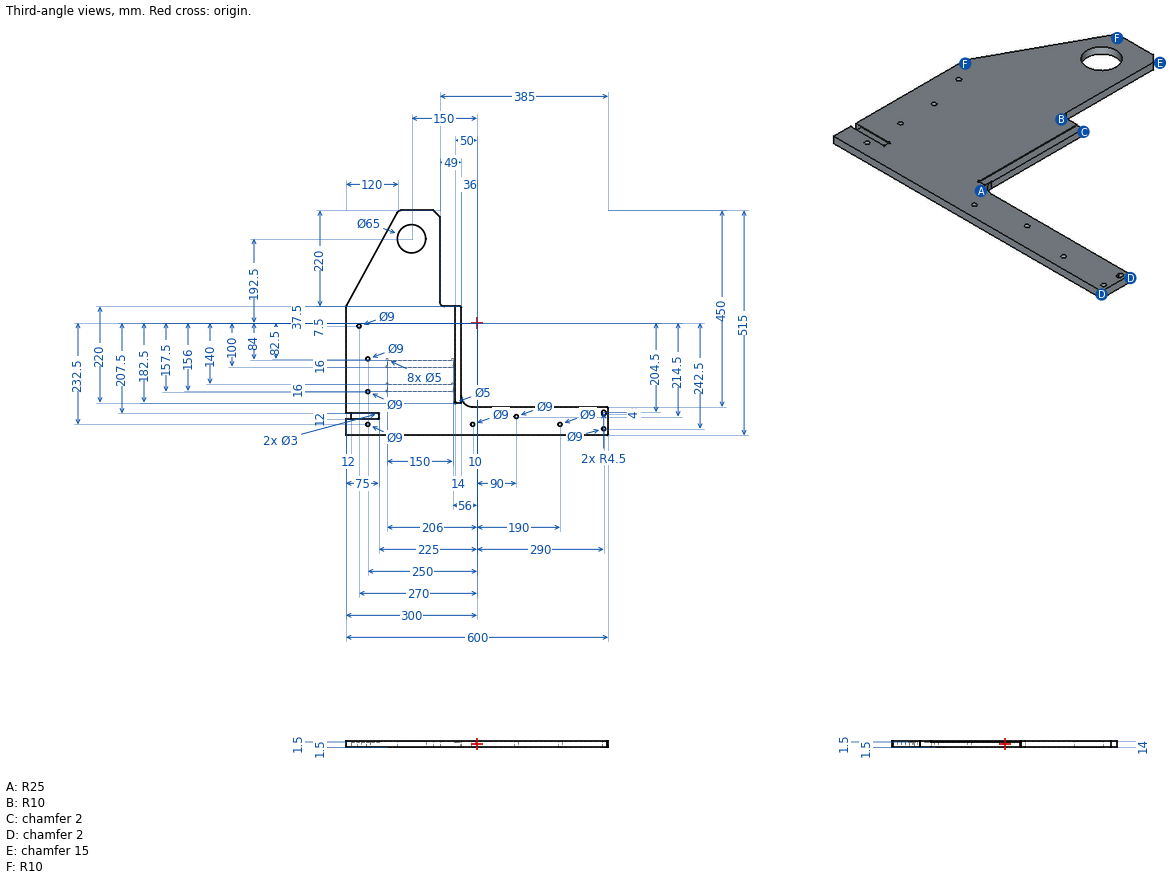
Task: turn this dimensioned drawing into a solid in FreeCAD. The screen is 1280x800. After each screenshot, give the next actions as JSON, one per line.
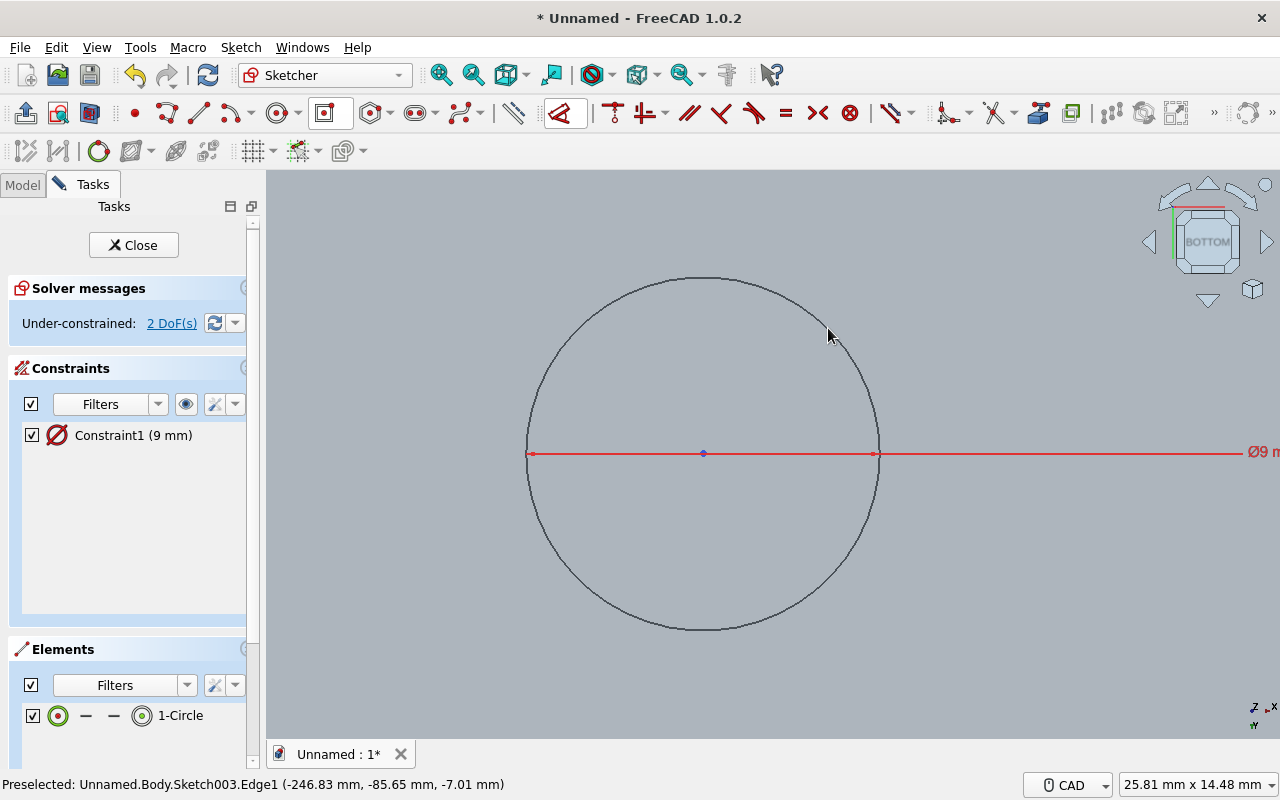
{"action": "left_click", "coordinate": [703, 454]}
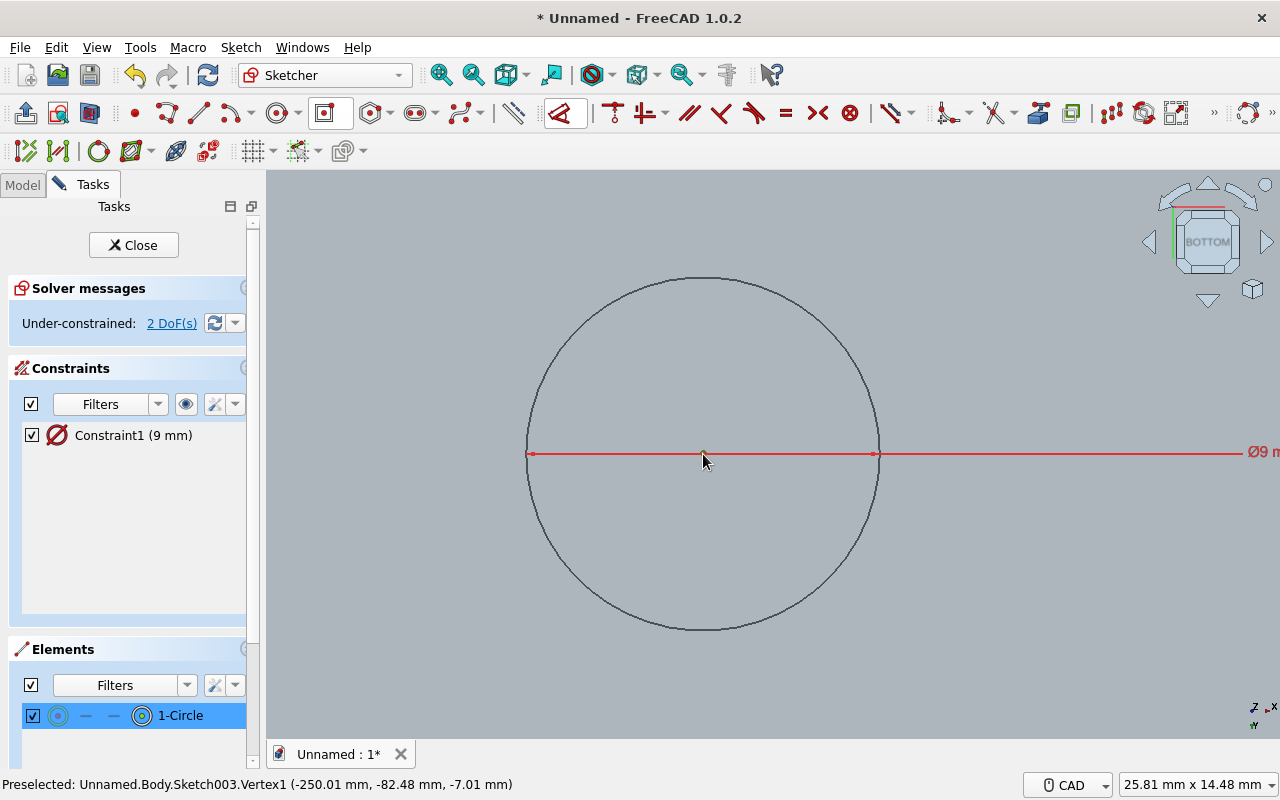
{"action": "left_click", "coordinate": [582, 114]}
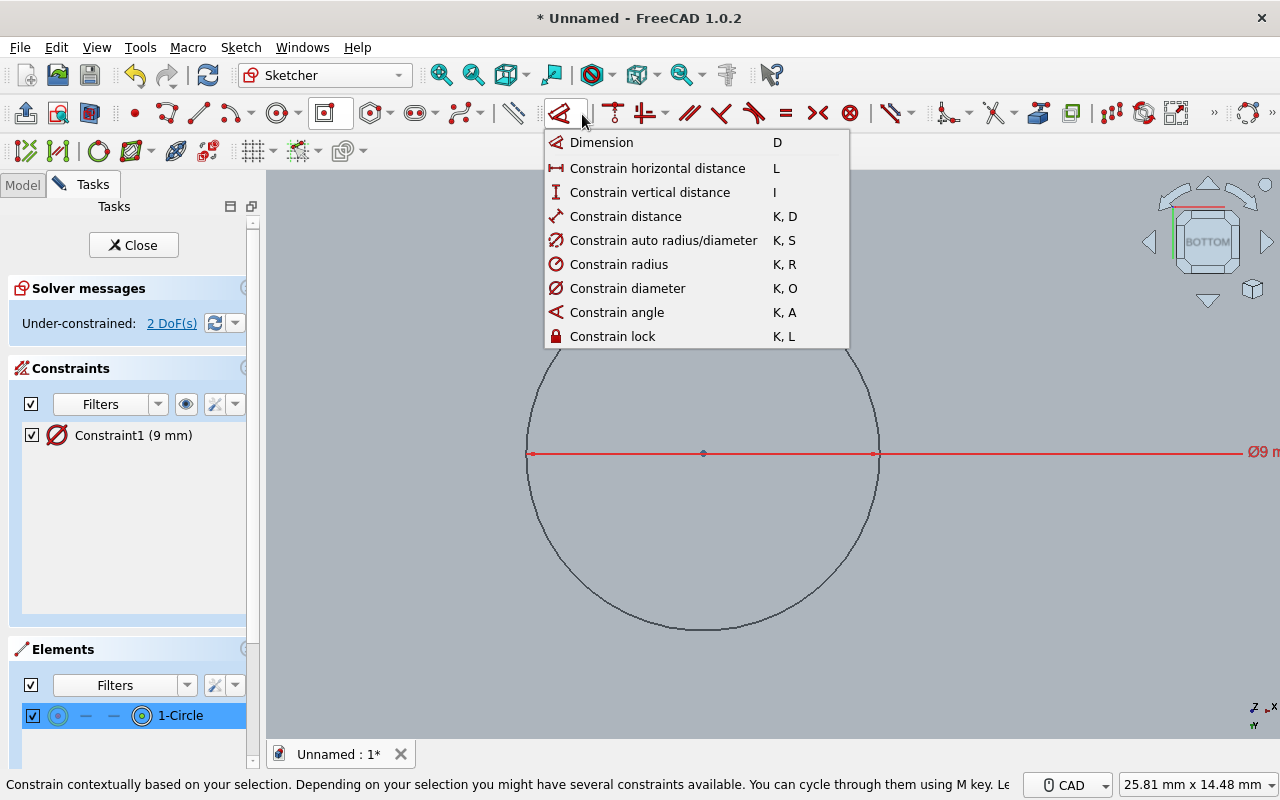
{"action": "left_click", "coordinate": [697, 168]}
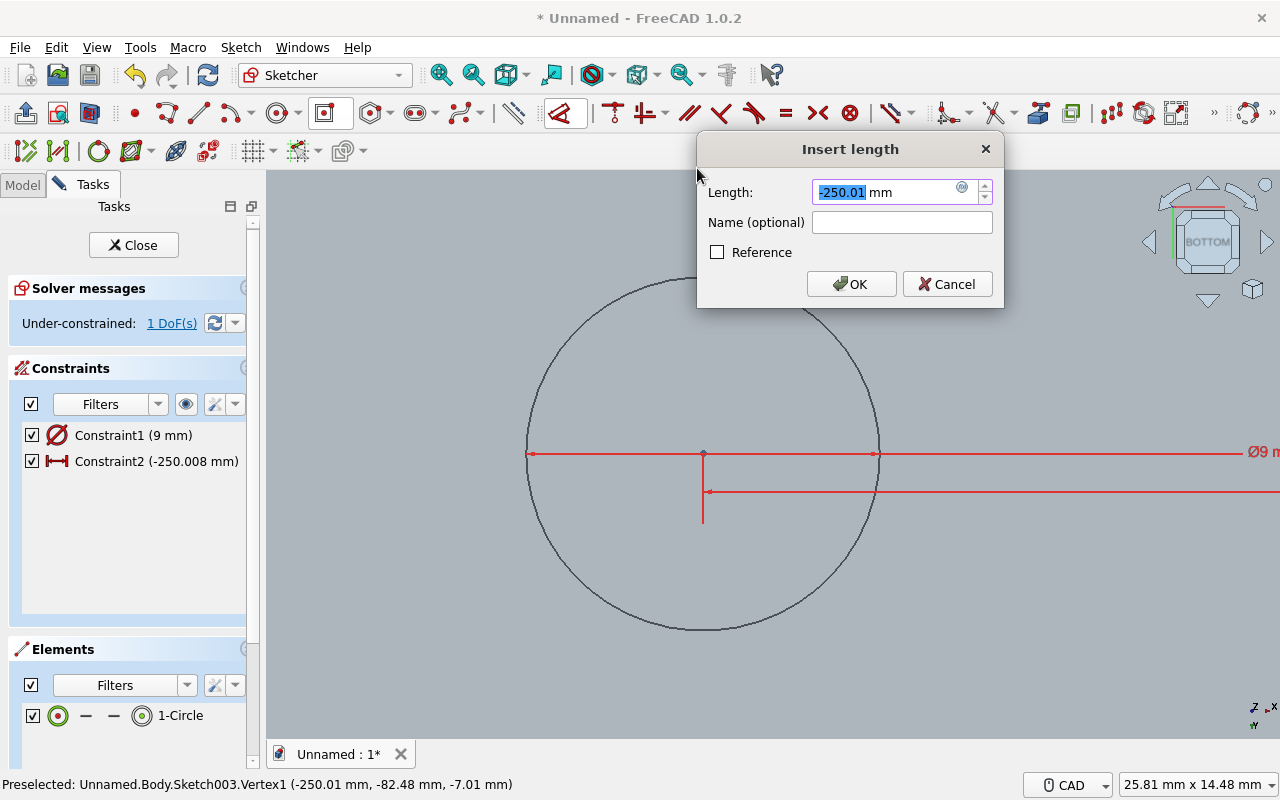
{"action": "type", "text": "-250"}
{"action": "key", "text": "Return"}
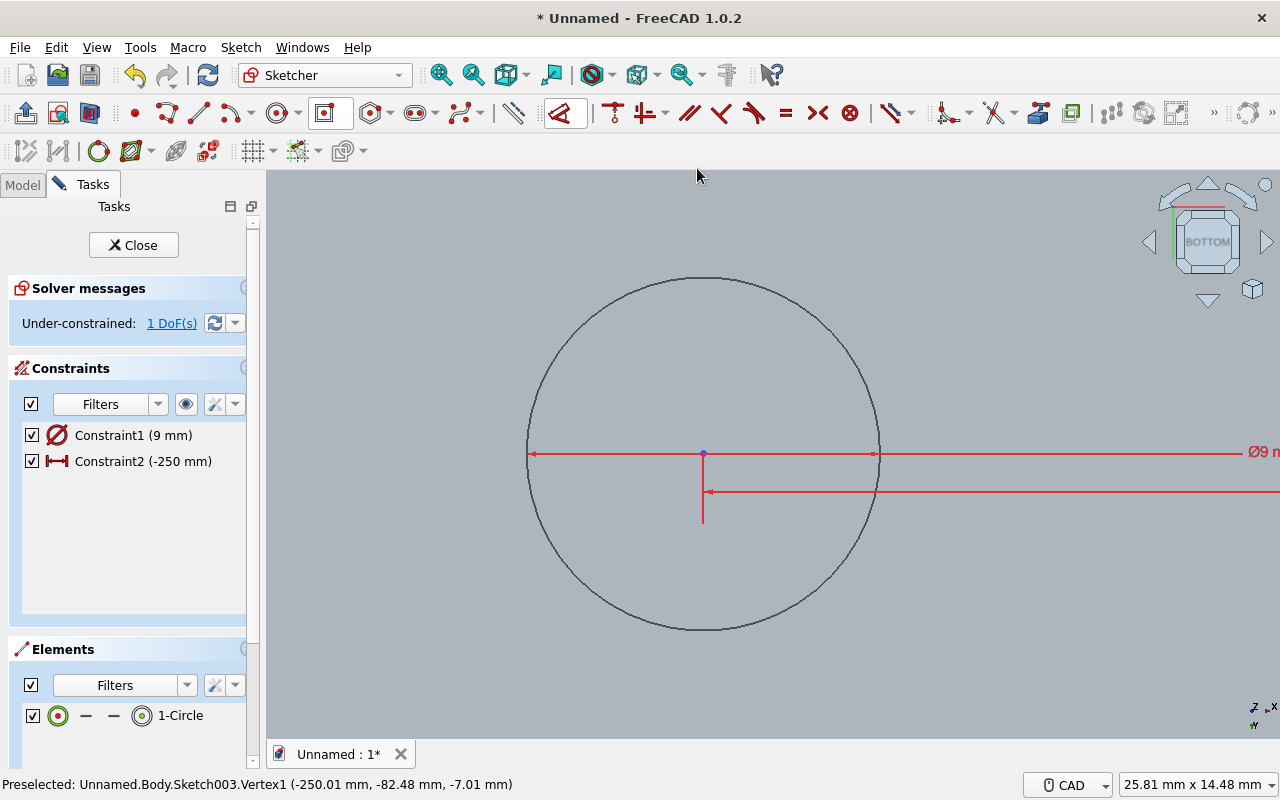
{"action": "left_click", "coordinate": [703, 454]}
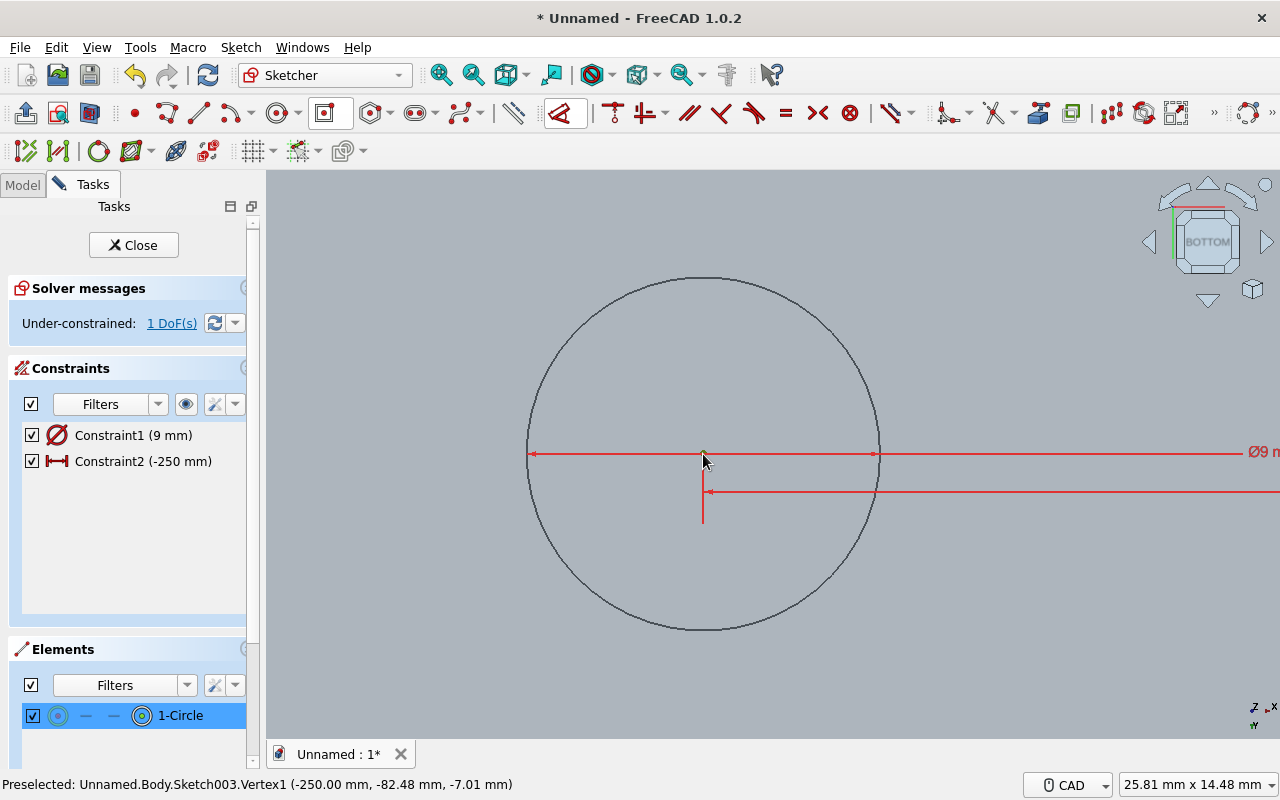
{"action": "key", "text": "i"}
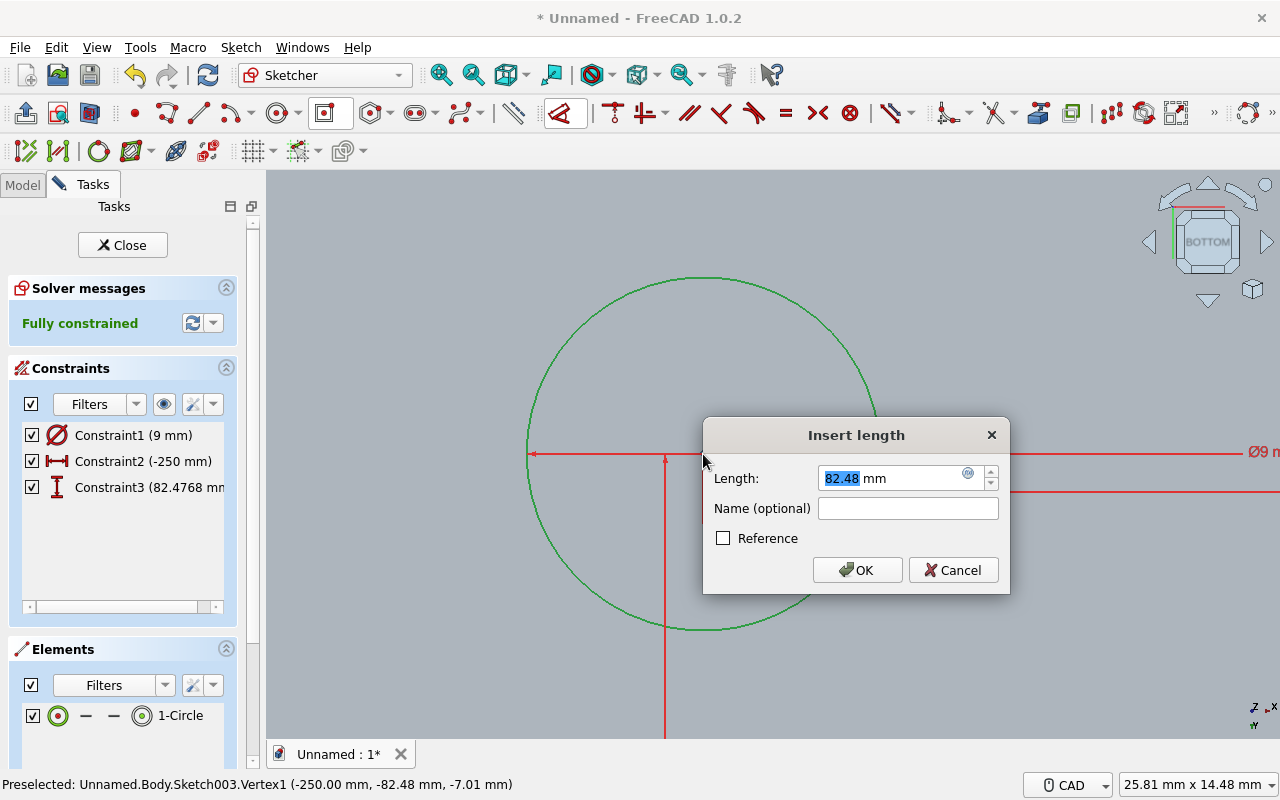
{"action": "type", "text": "82.5"}
{"action": "key", "text": "Return"}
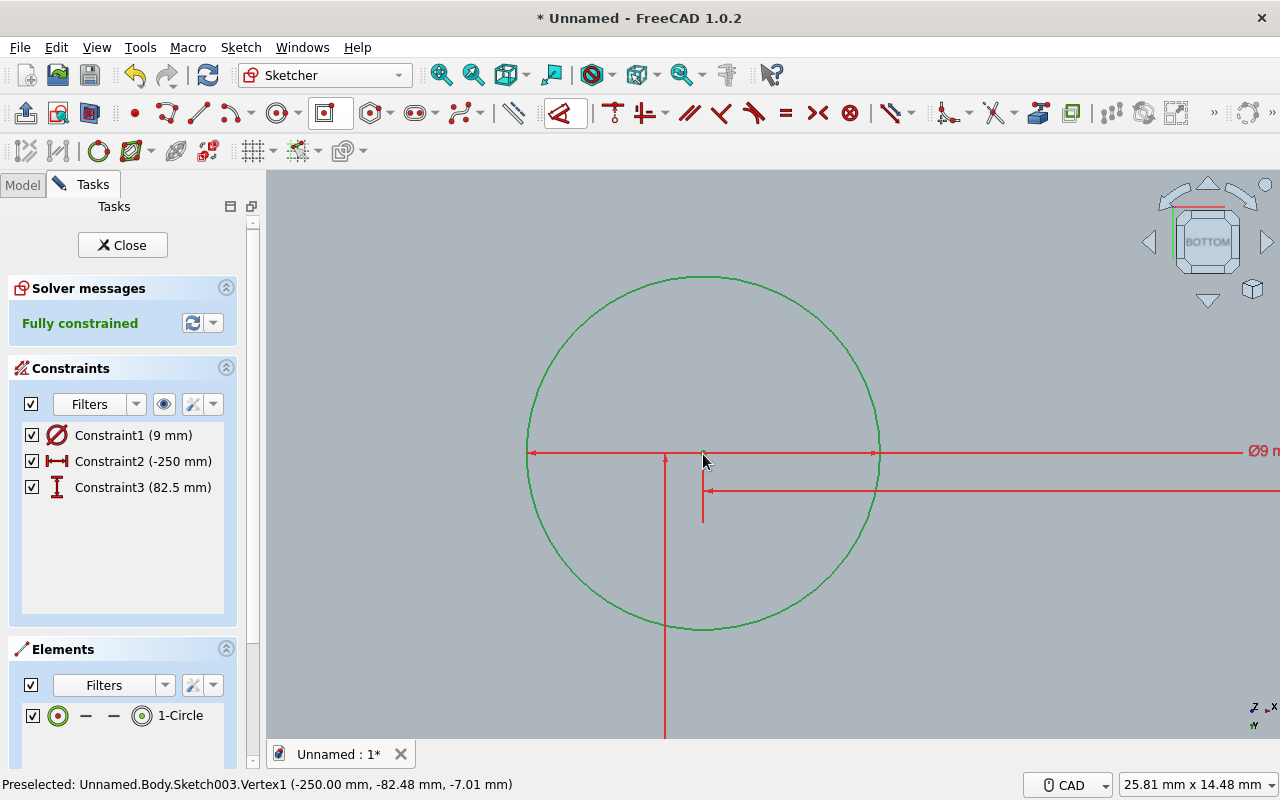
{"action": "left_click", "coordinate": [123, 245]}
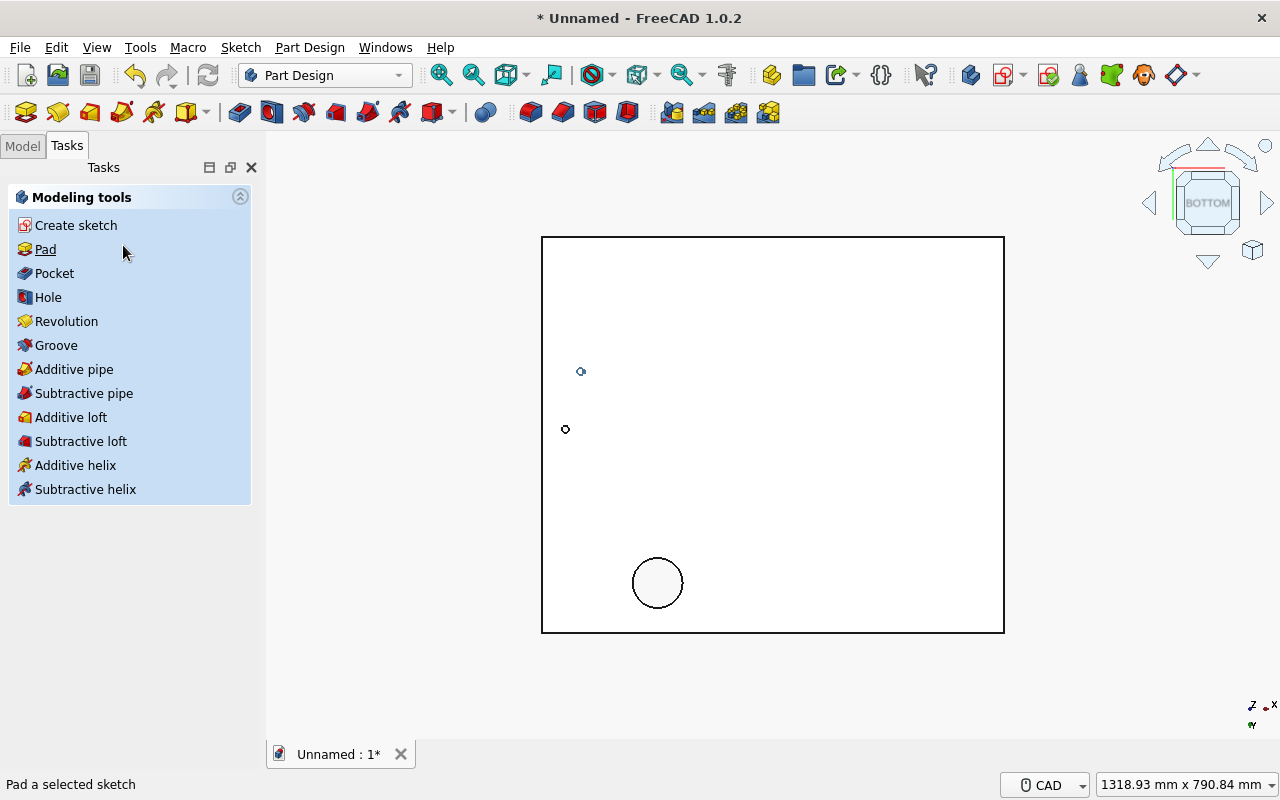
{"action": "left_click", "coordinate": [240, 112]}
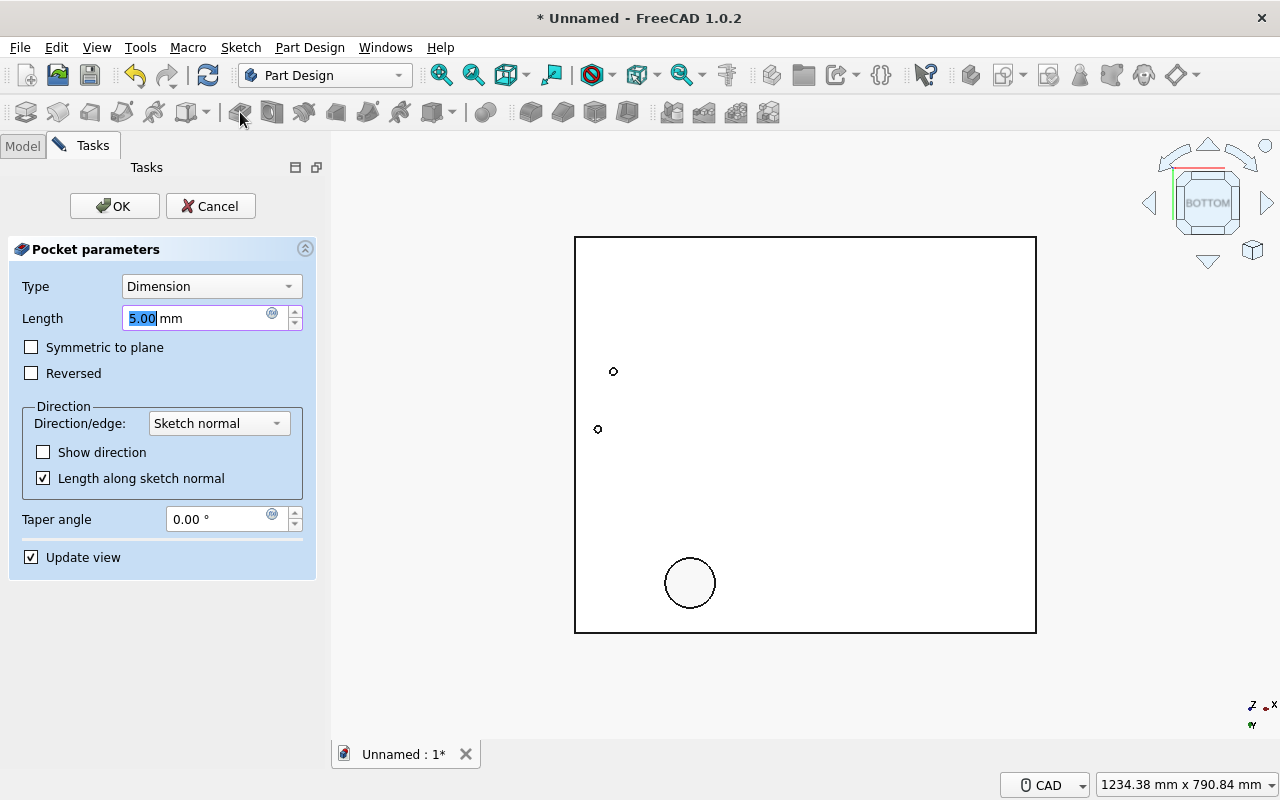
{"action": "left_click", "coordinate": [212, 286]}